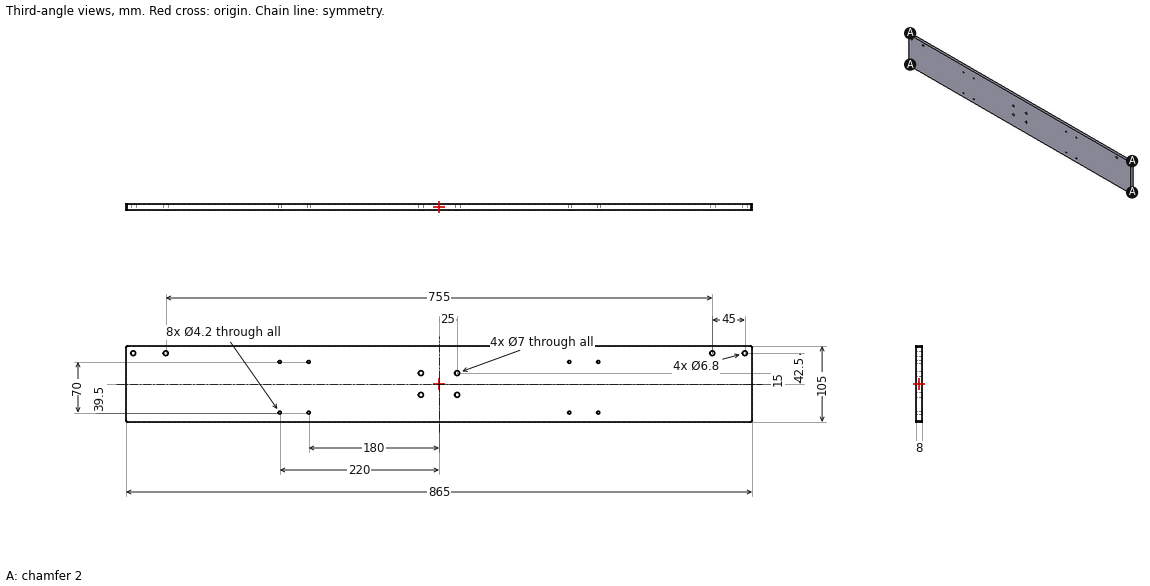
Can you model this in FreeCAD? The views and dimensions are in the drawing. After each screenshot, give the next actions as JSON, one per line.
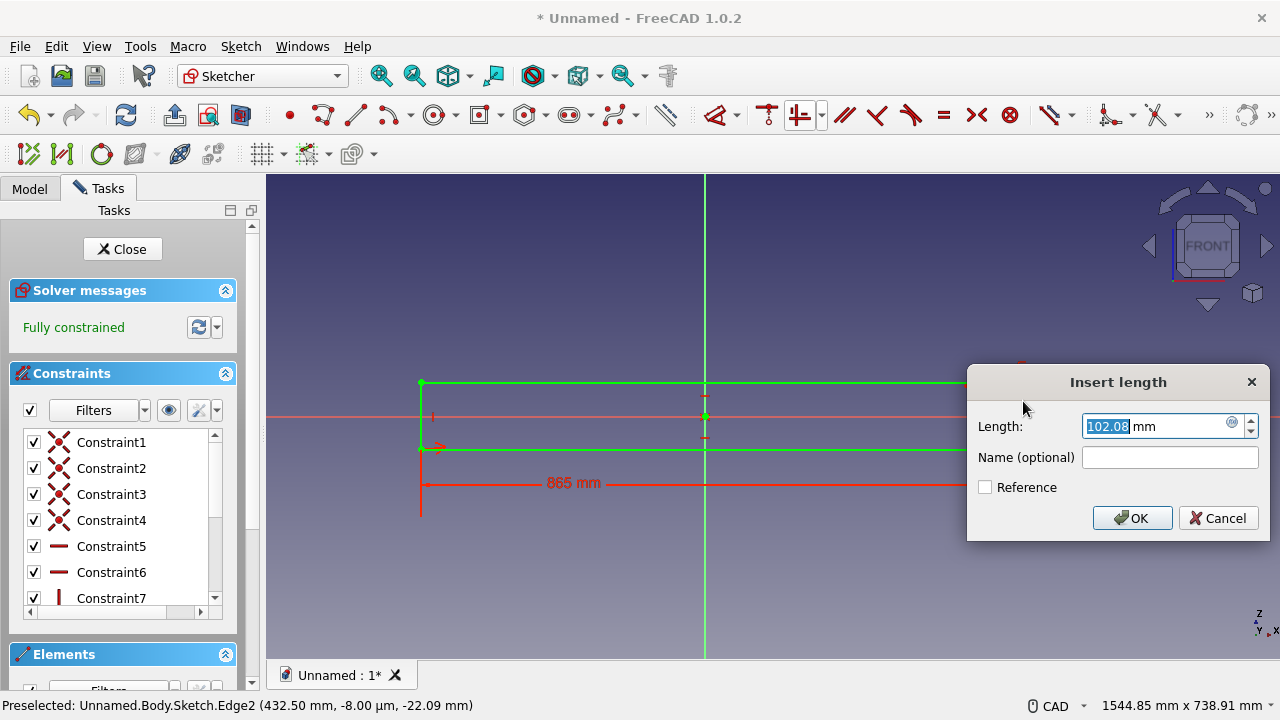
{"action": "type", "text": "105"}
{"action": "key", "text": "Return"}
{"action": "key", "text": "Escape"}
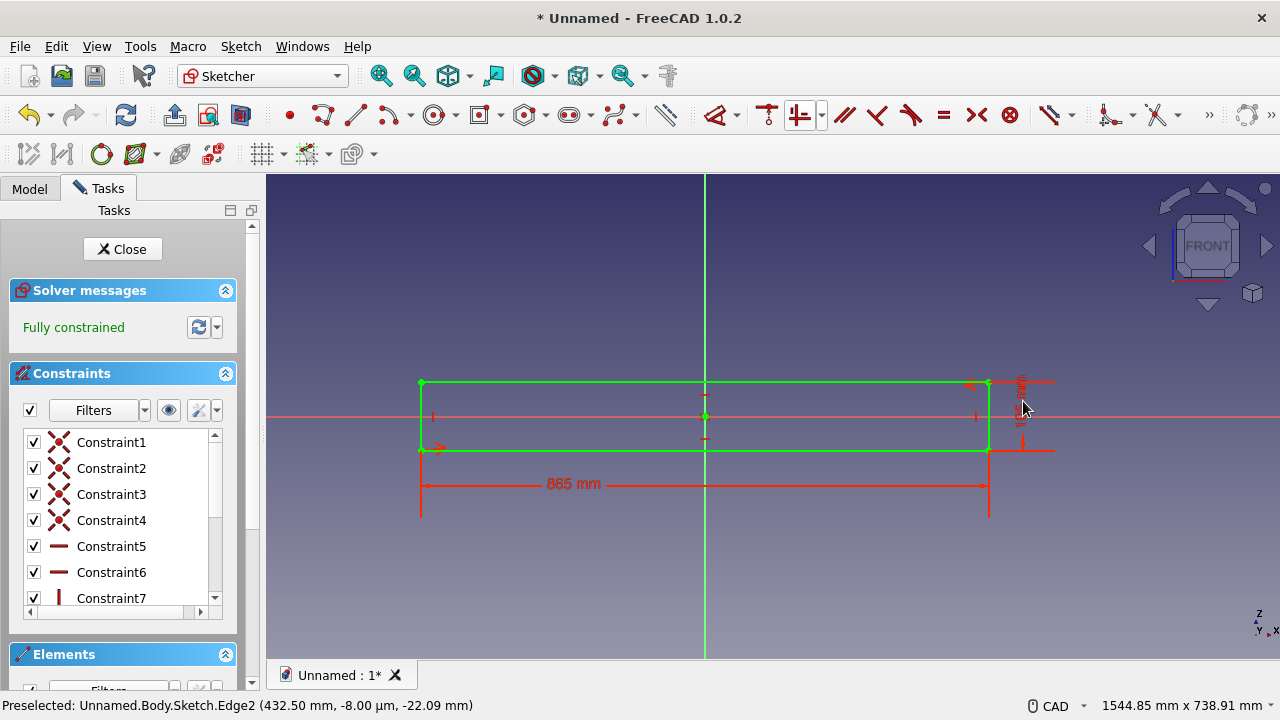
{"action": "left_click", "coordinate": [123, 249]}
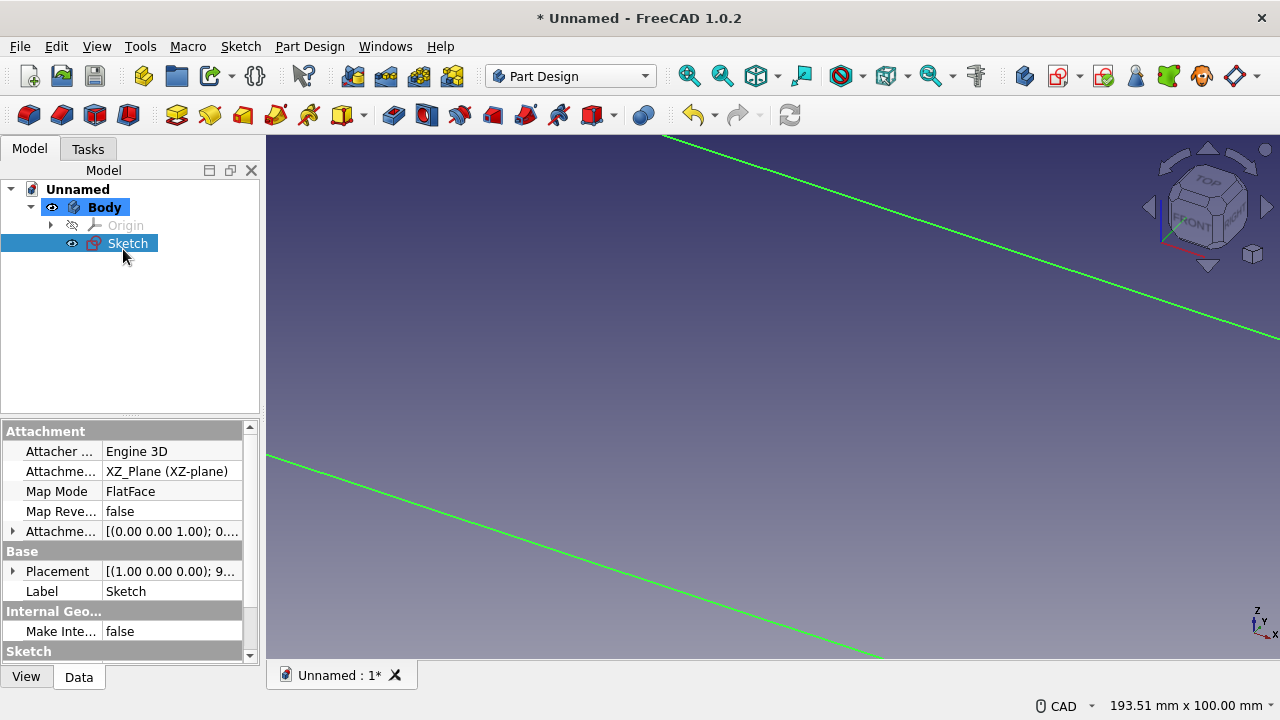
{"action": "left_click", "coordinate": [177, 116]}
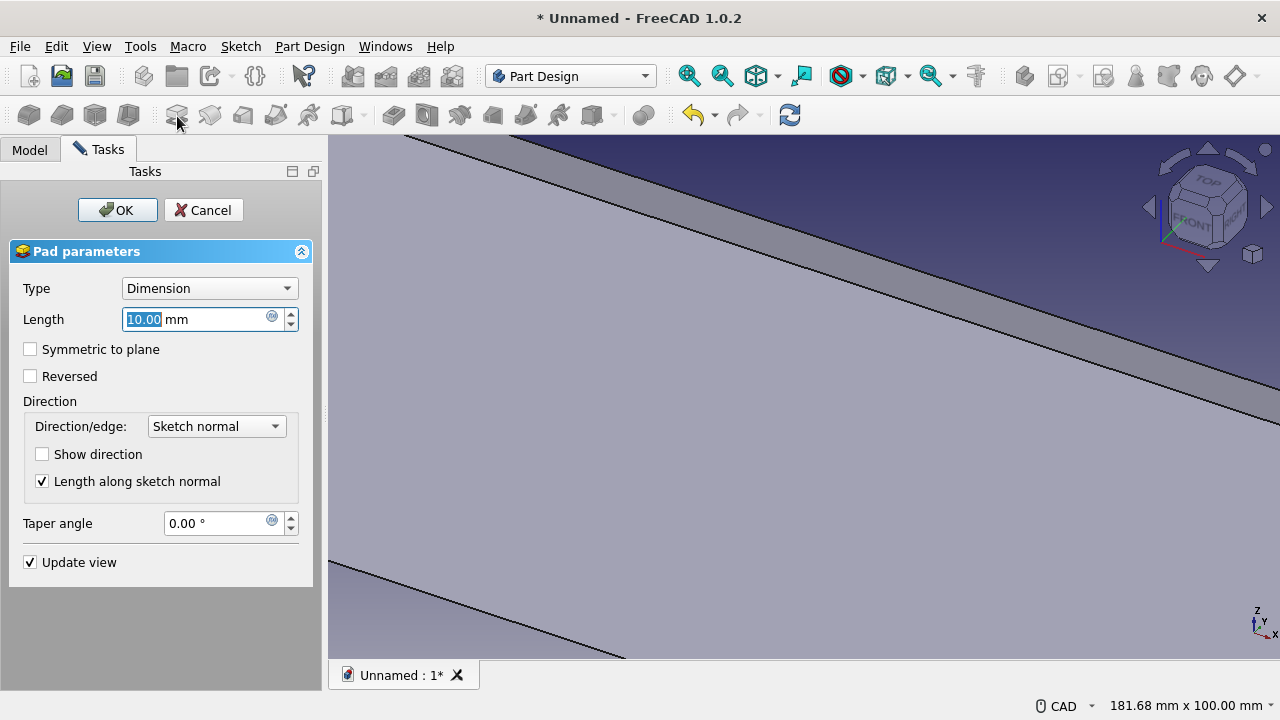
{"action": "type", "text": "8"}
{"action": "key", "text": "Tab"}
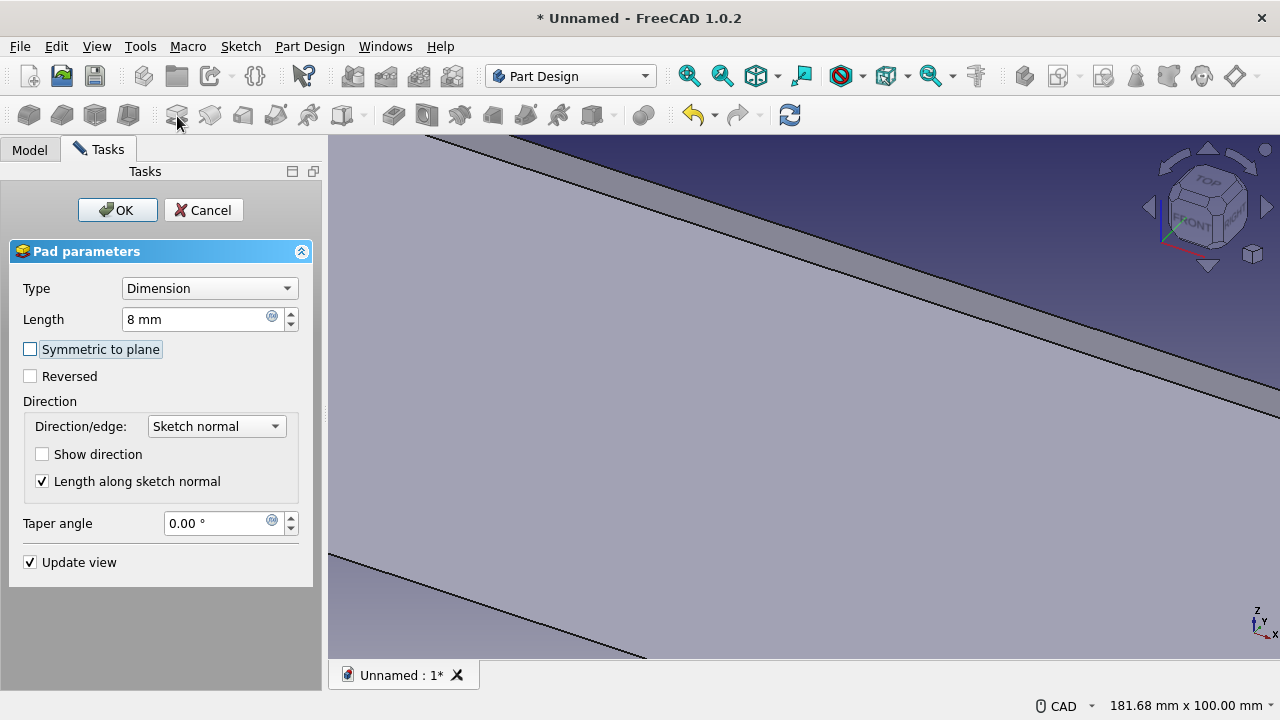
{"action": "left_click", "coordinate": [31, 349]}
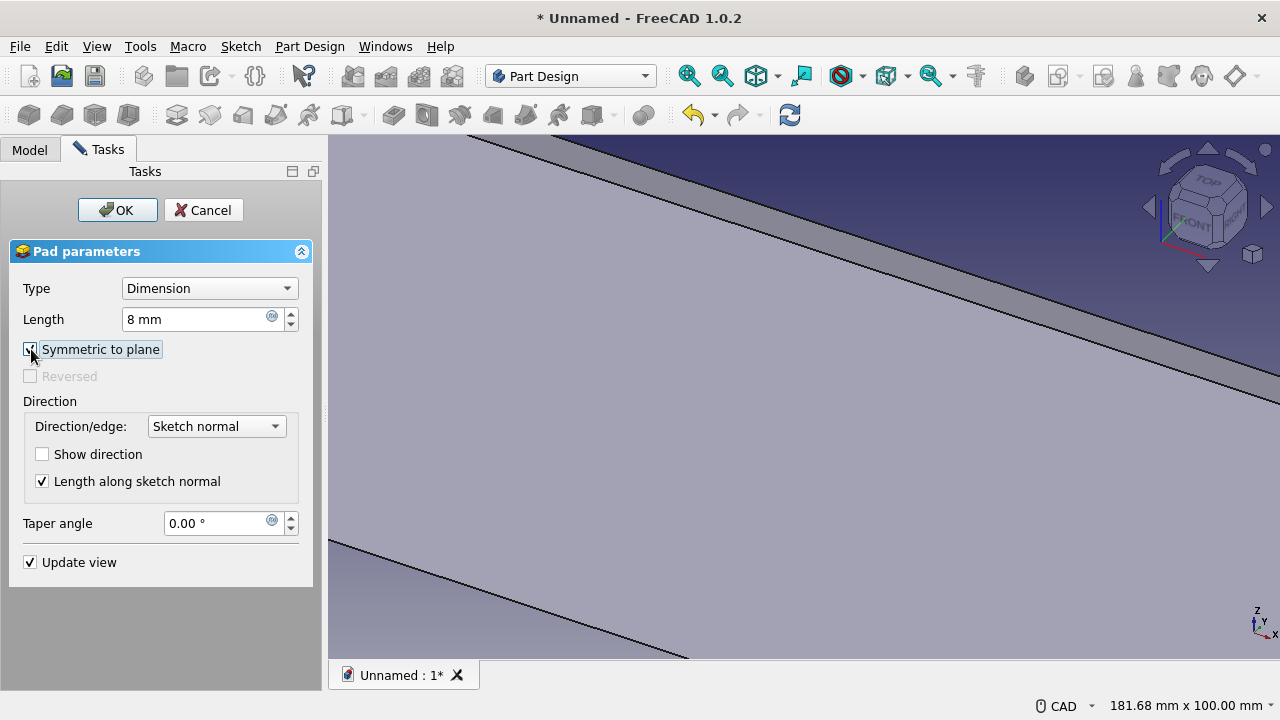
{"action": "left_click", "coordinate": [118, 210]}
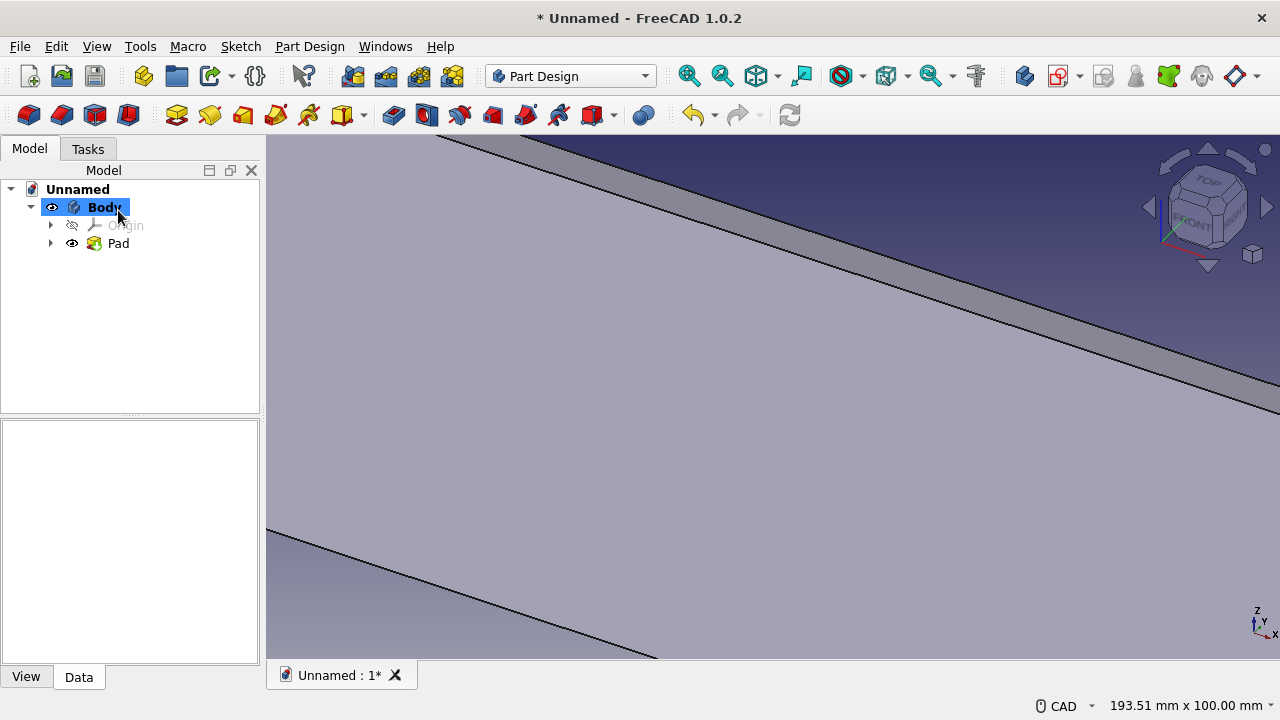
{"action": "key", "text": "v f"}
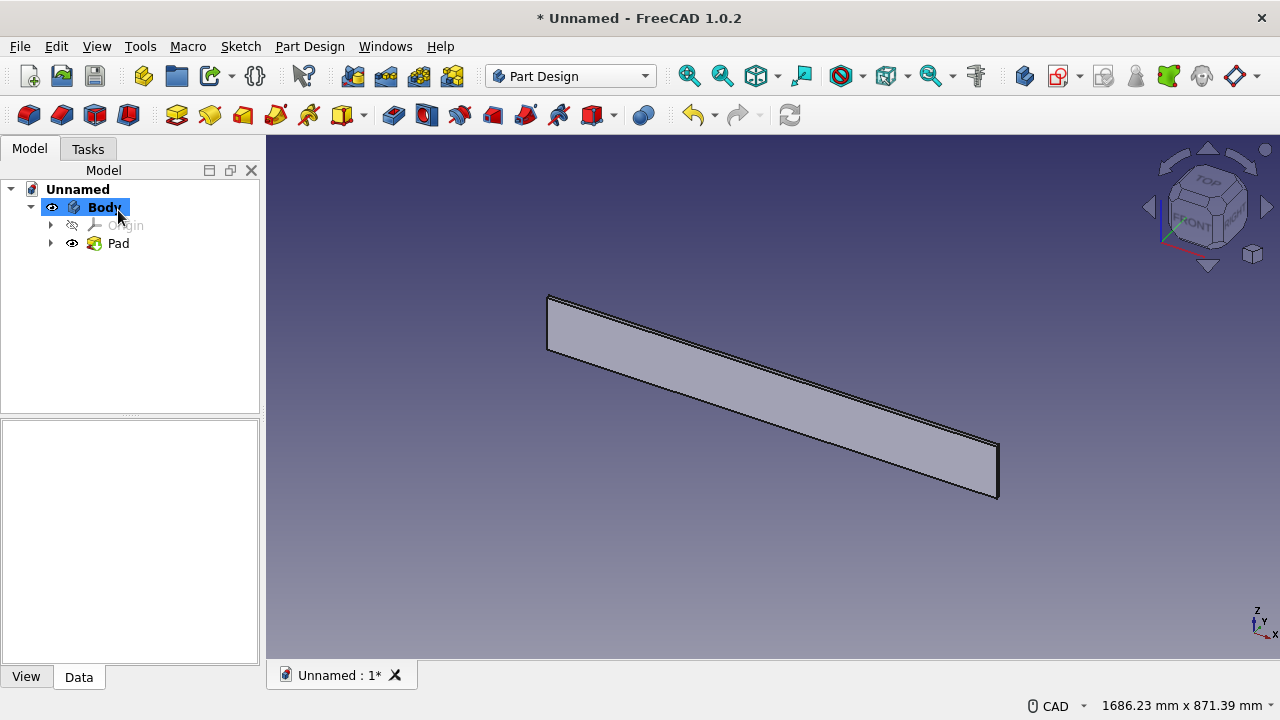
{"action": "scroll", "coordinate": [998, 445], "scroll_direction": "up", "scroll_amount": 11}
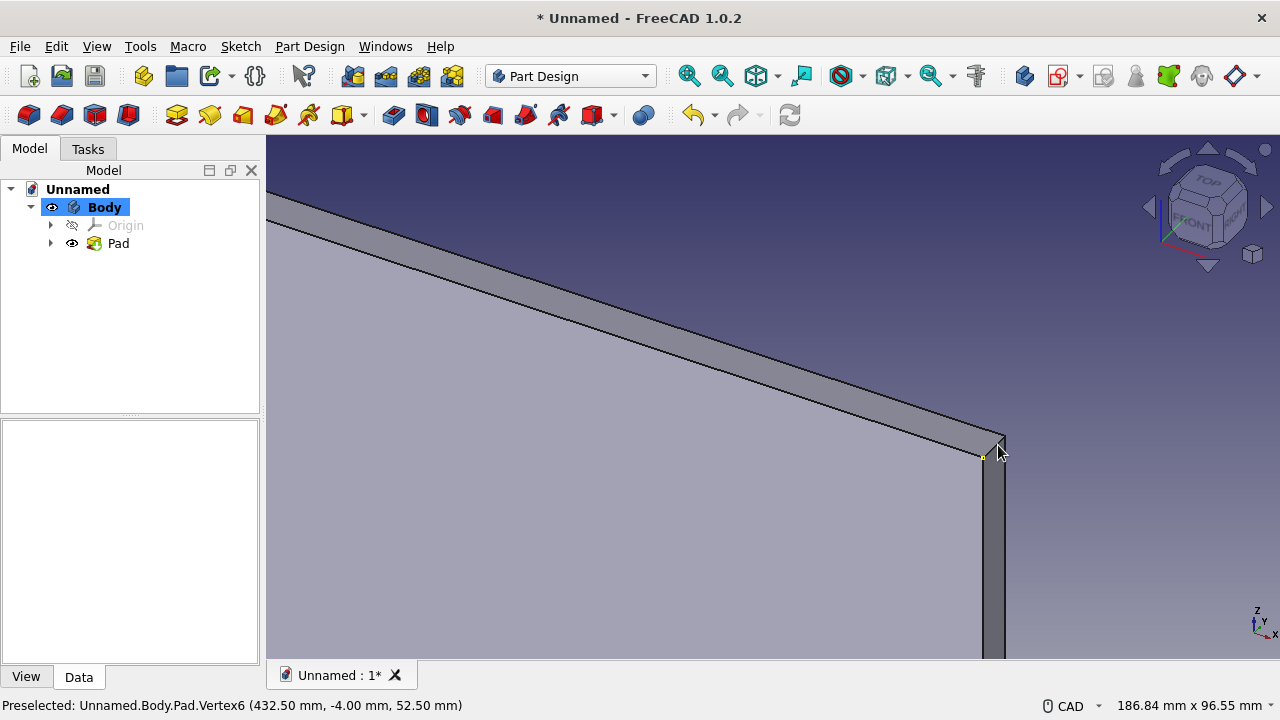
{"action": "left_click", "coordinate": [994, 446]}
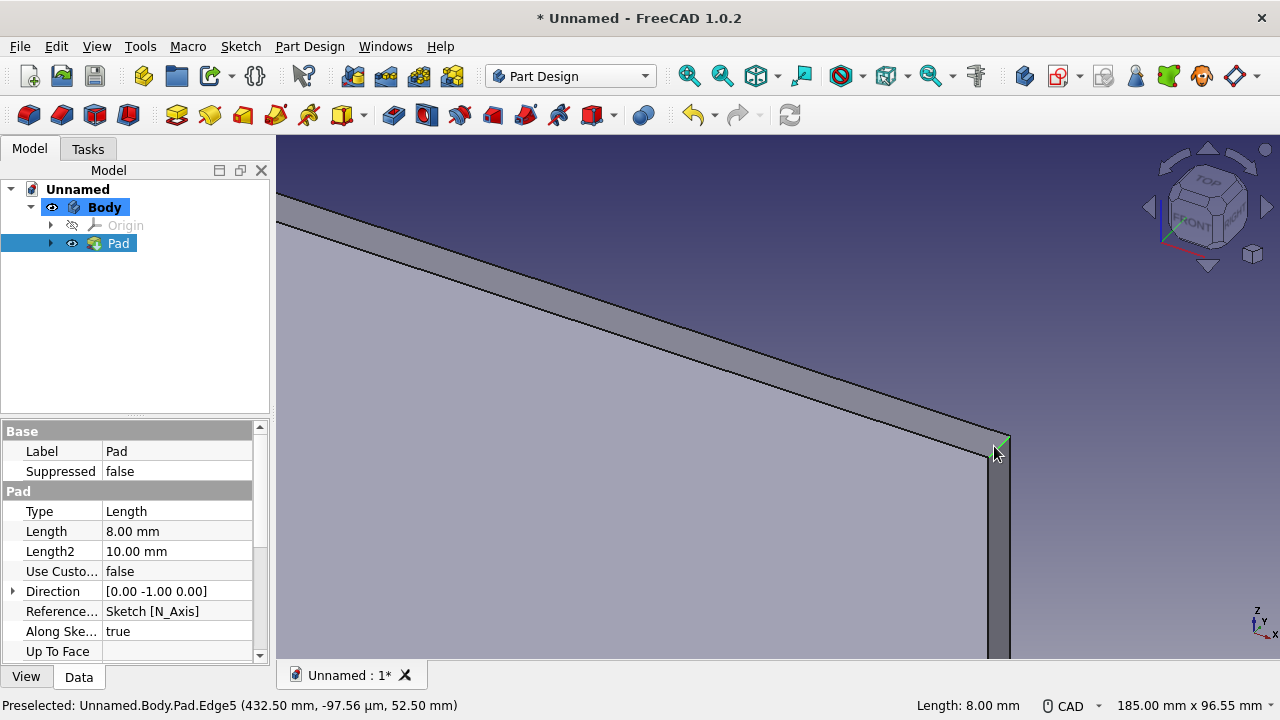
{"action": "key", "text": "v f"}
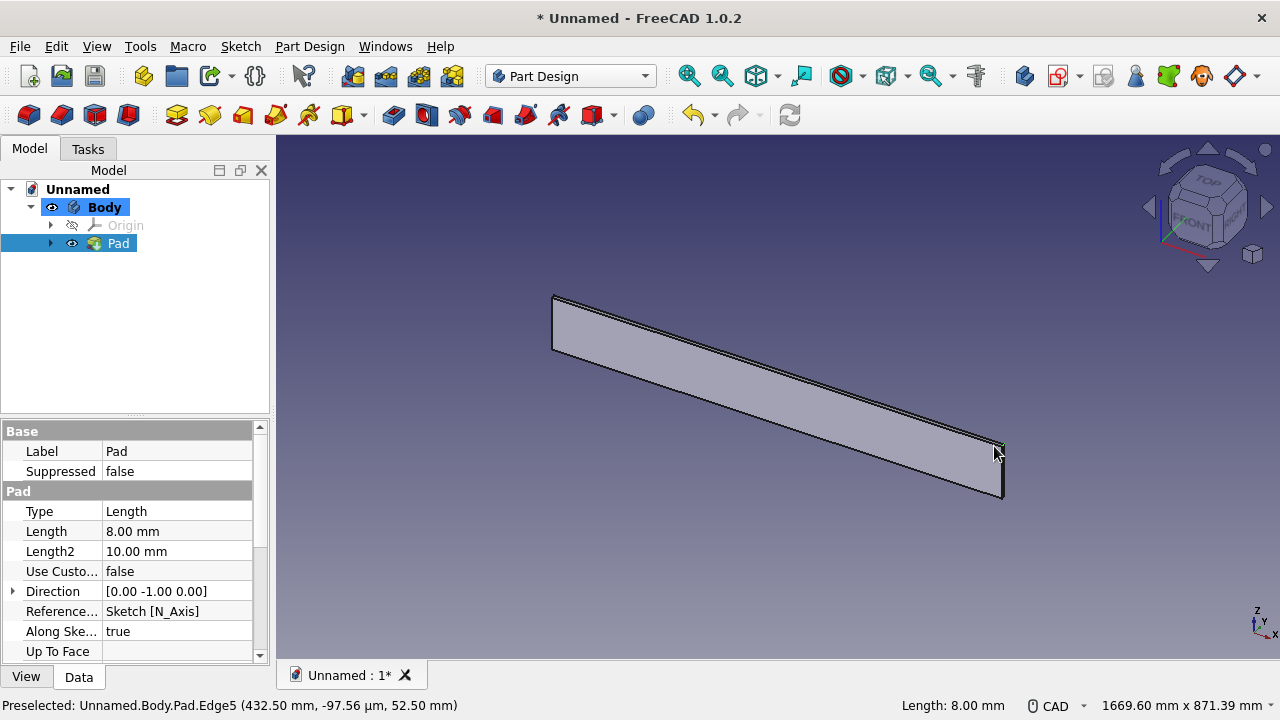
{"action": "key", "text": "0"}